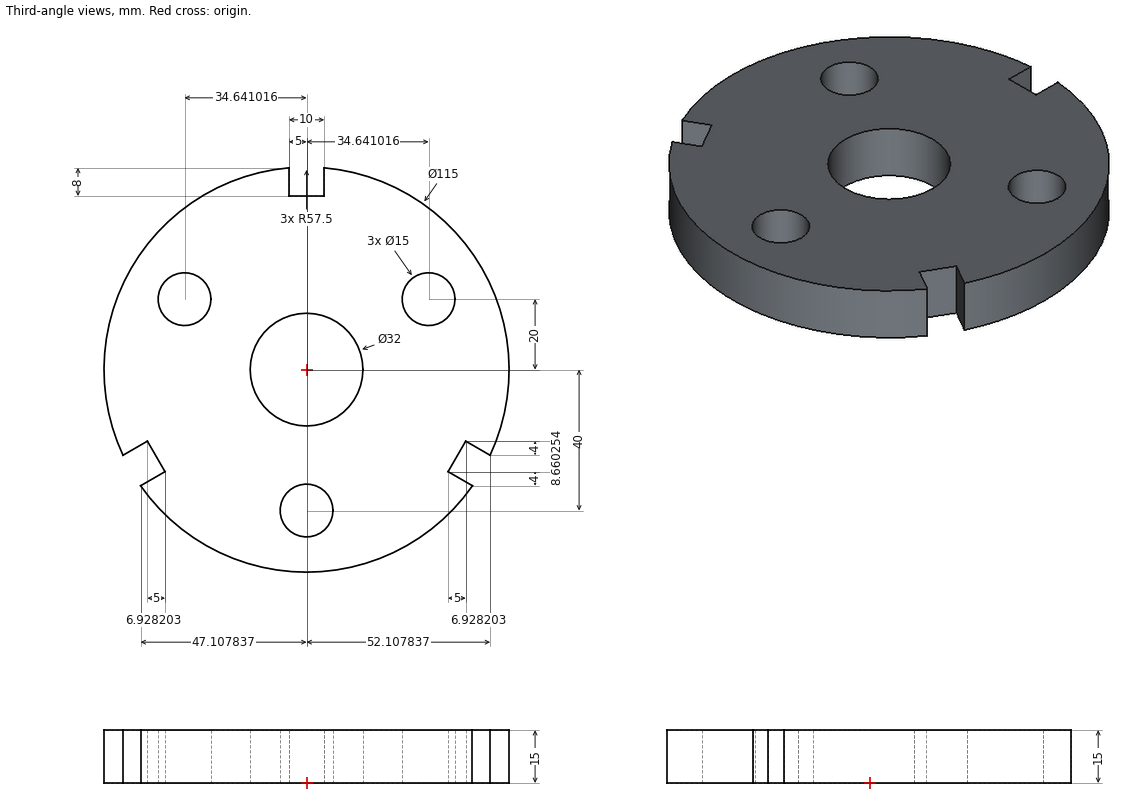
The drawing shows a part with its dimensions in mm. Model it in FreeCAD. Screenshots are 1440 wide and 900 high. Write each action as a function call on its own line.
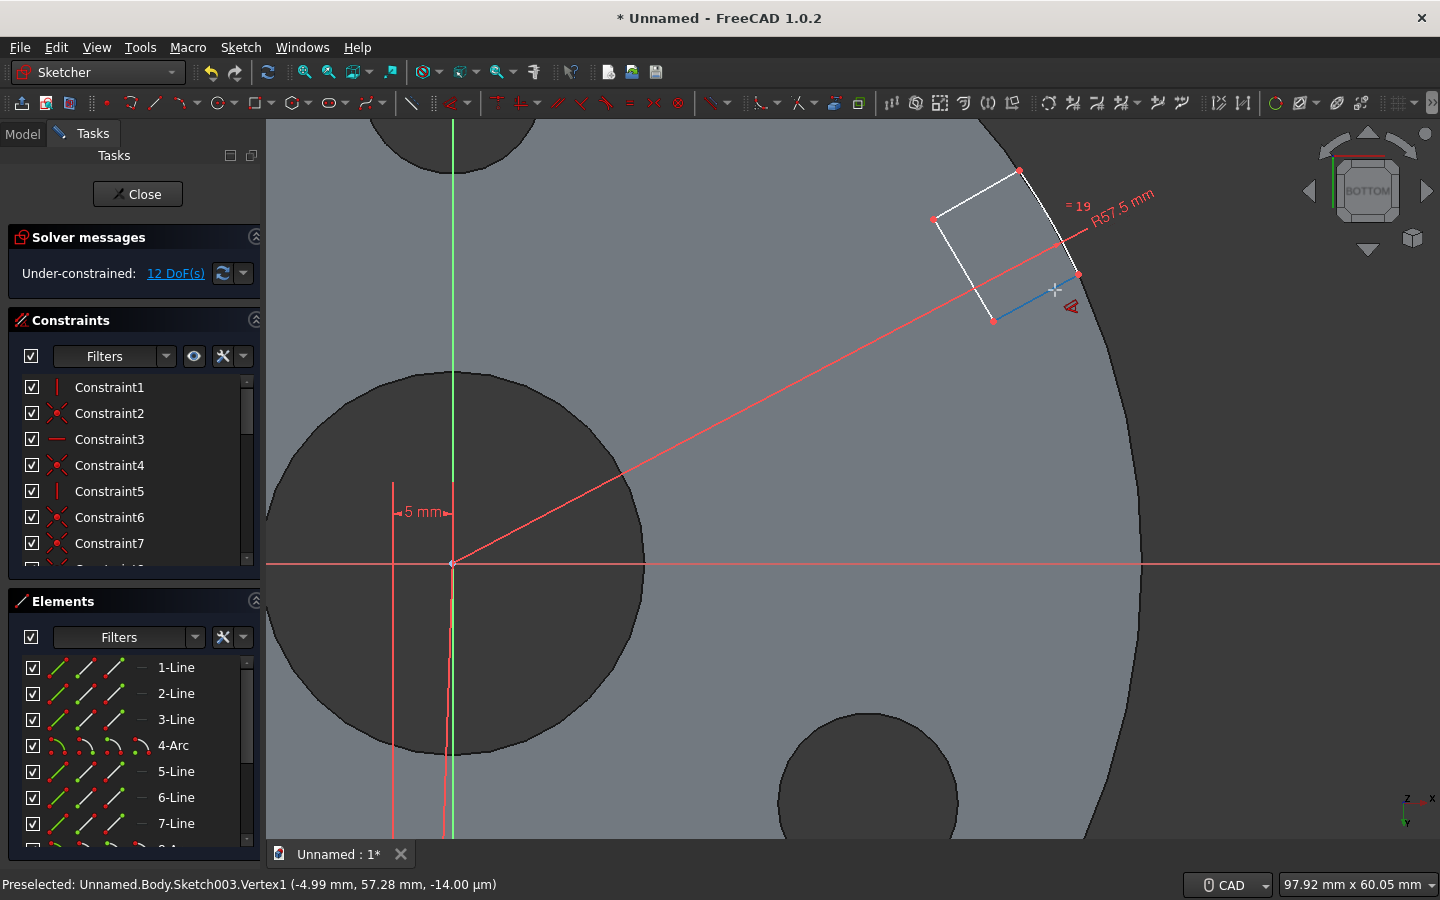
click(1053, 289)
click(1113, 298)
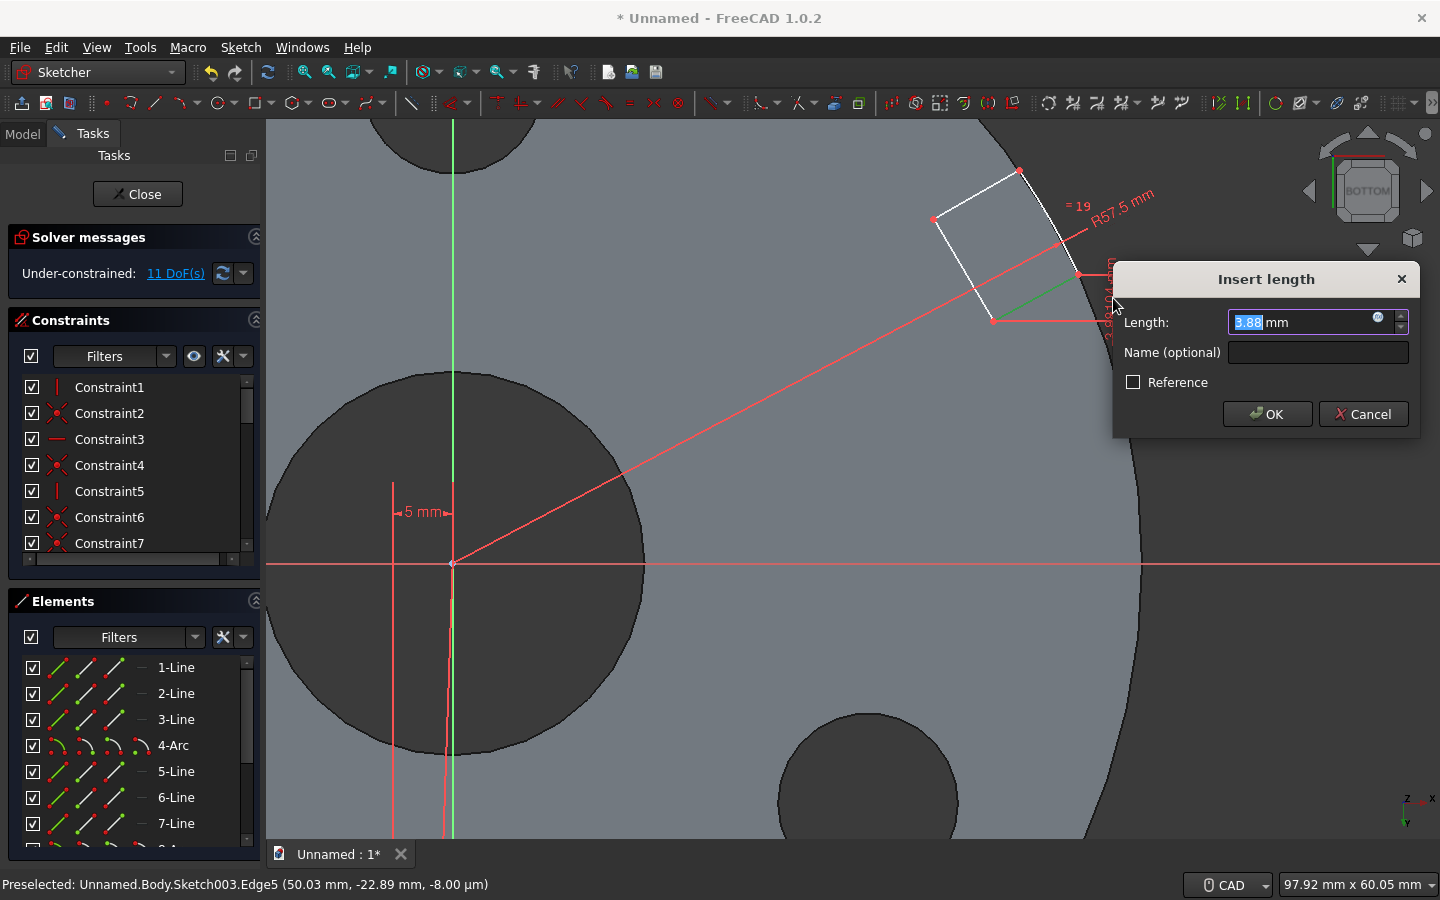
text(4)
key(Return)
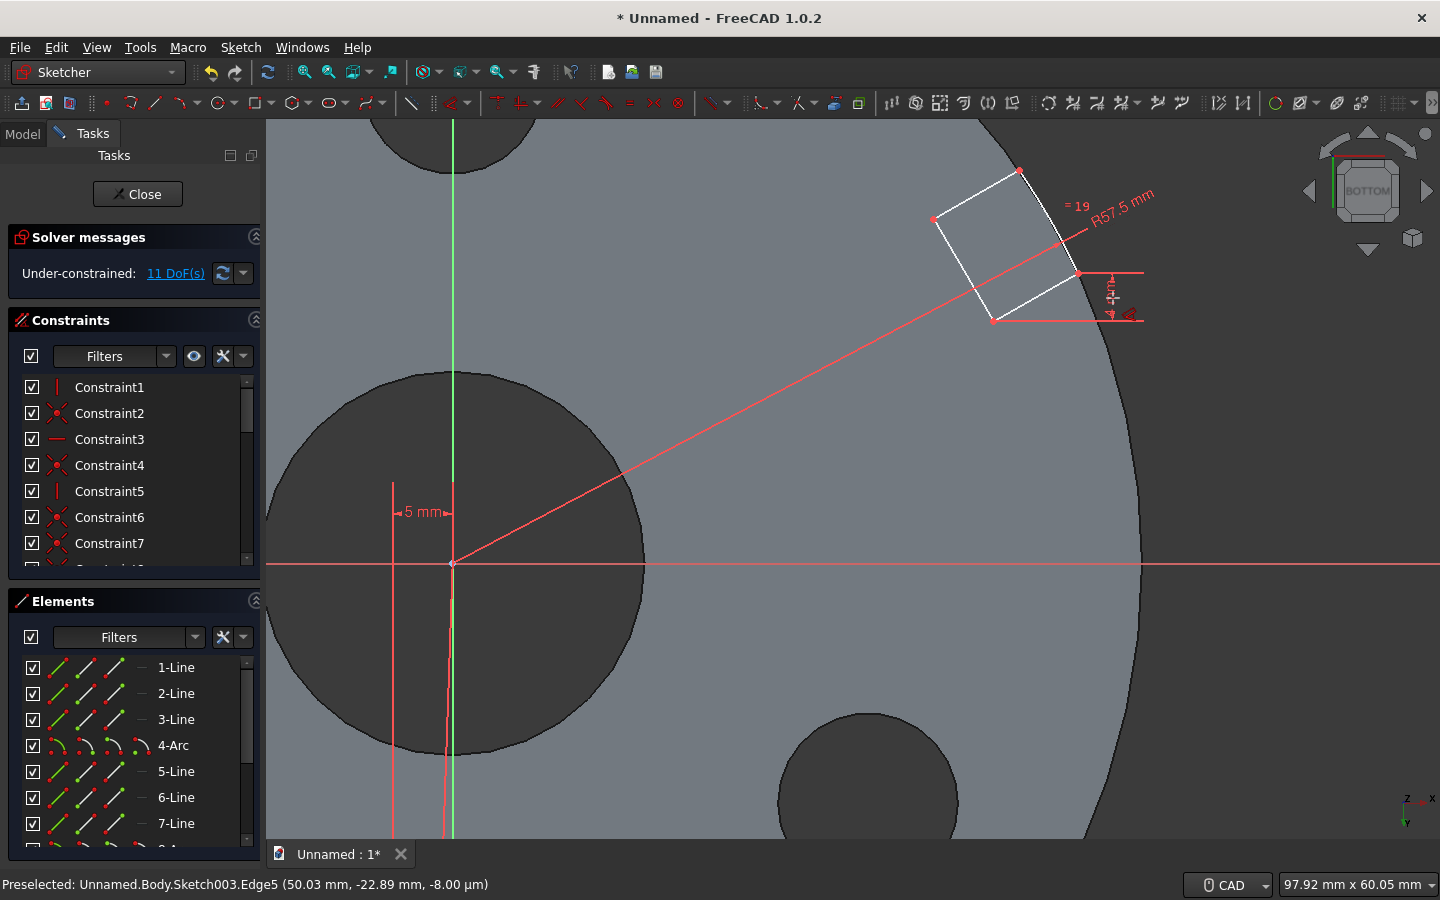
click(976, 291)
click(964, 185)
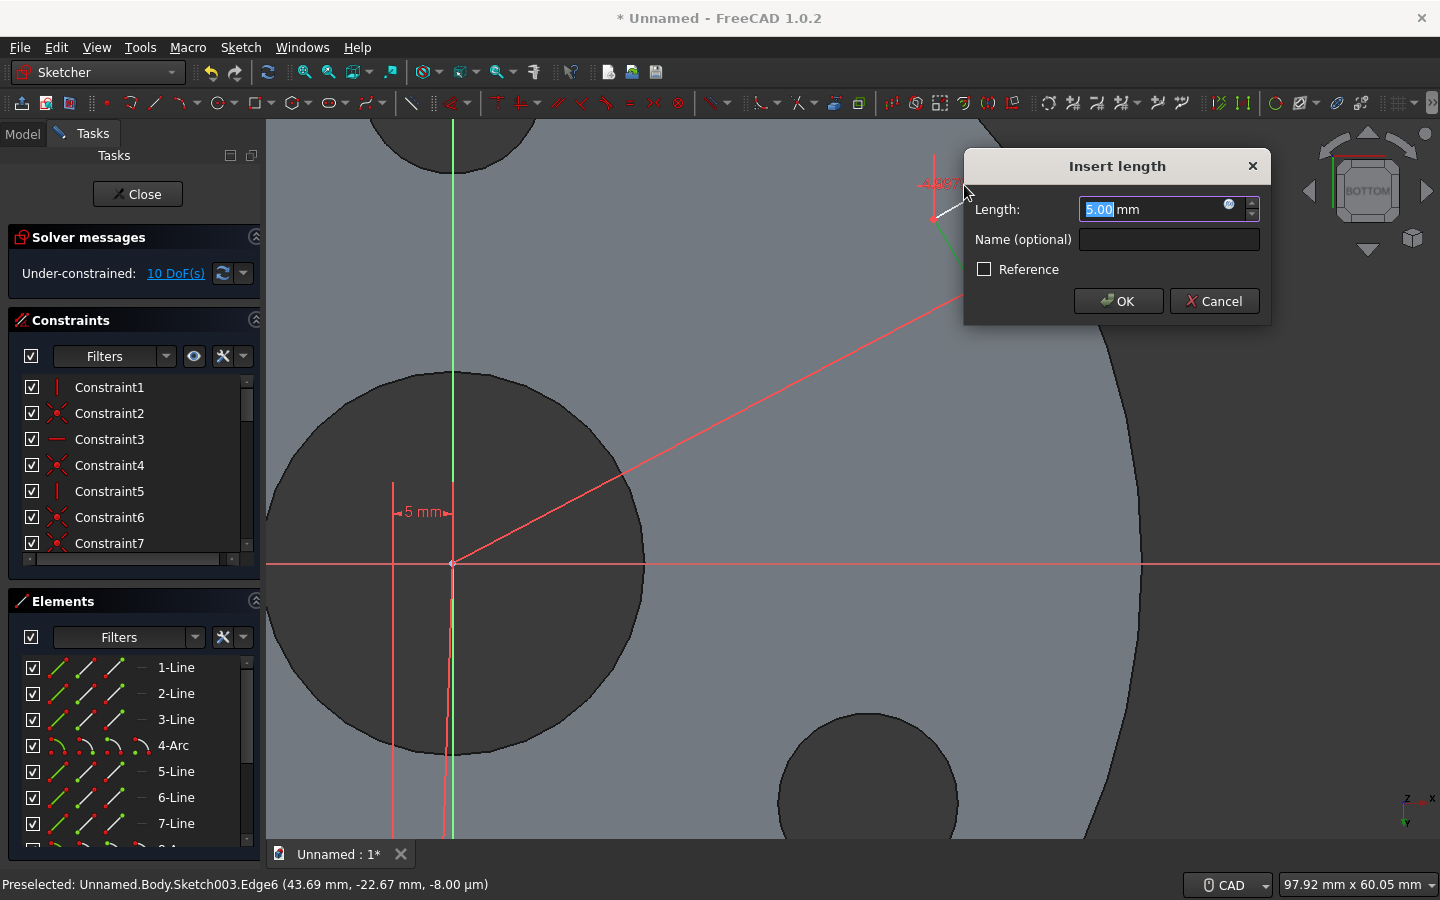
text(5)
key(Return)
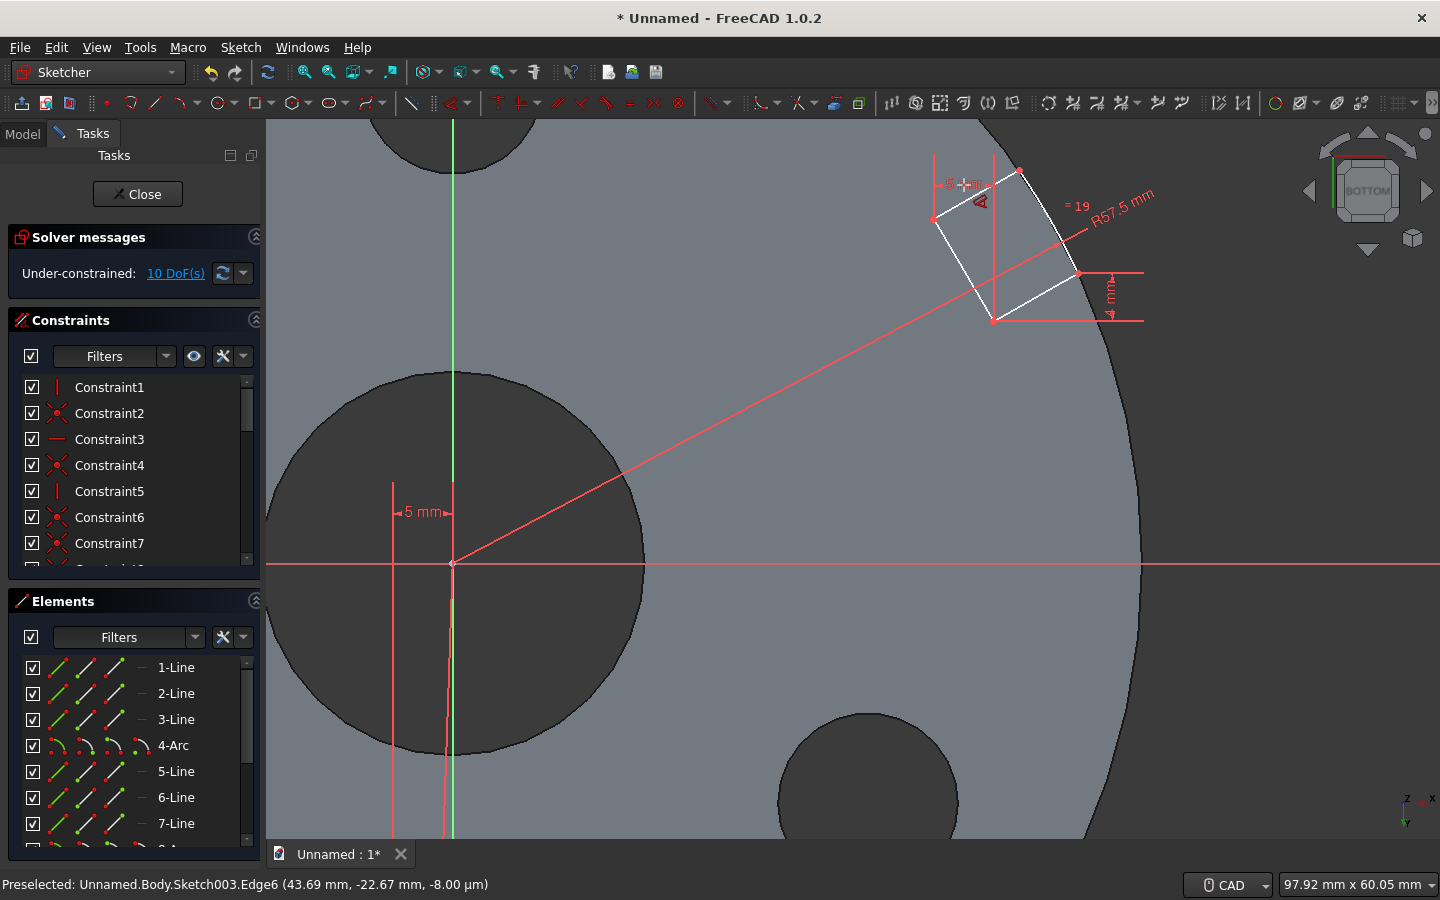
click(959, 204)
click(1053, 184)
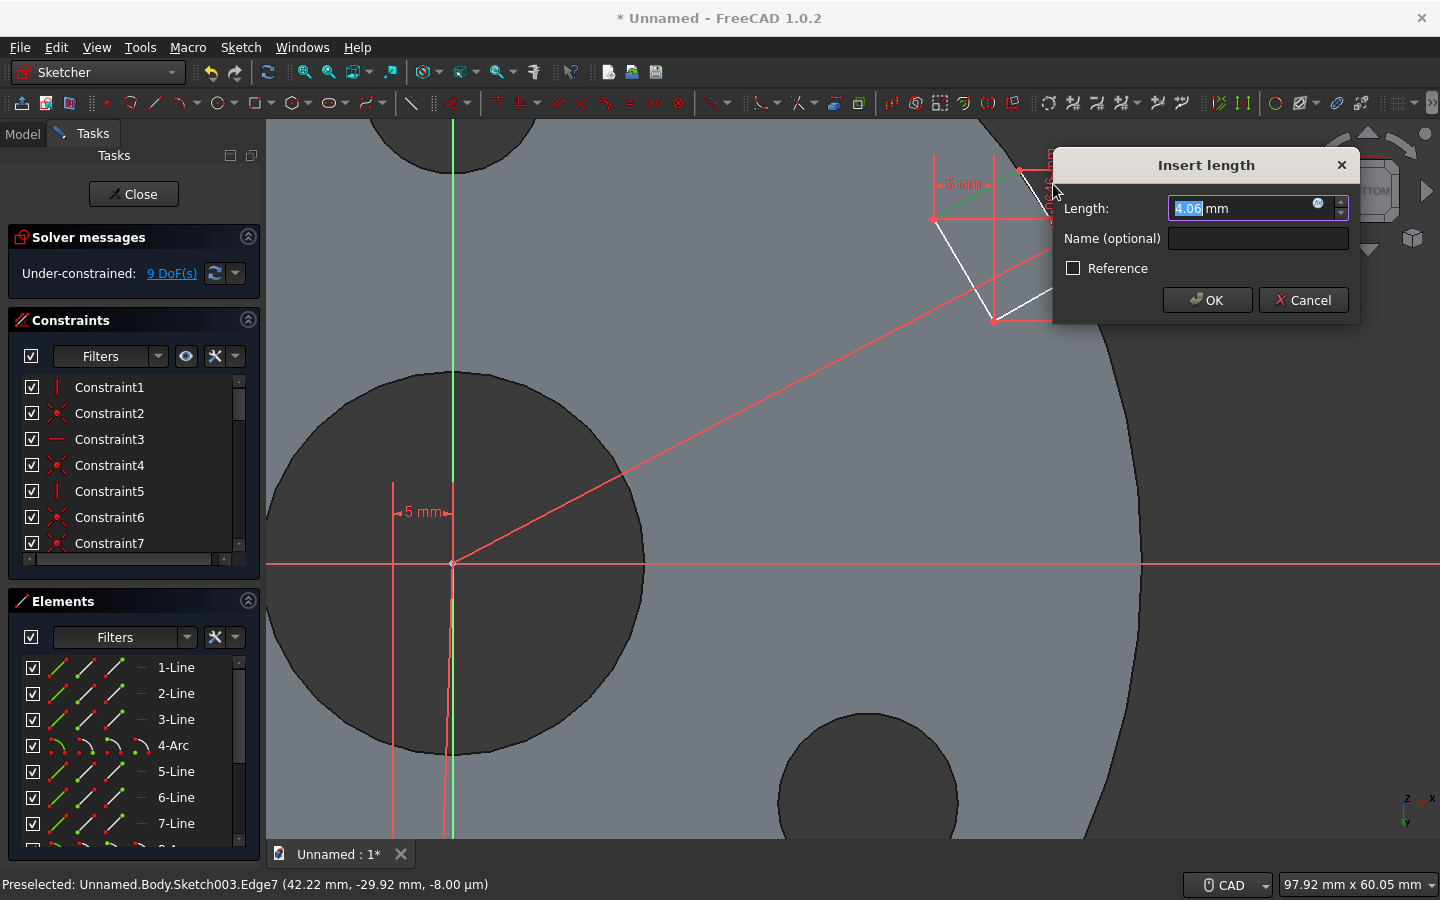
text(4)
key(Return)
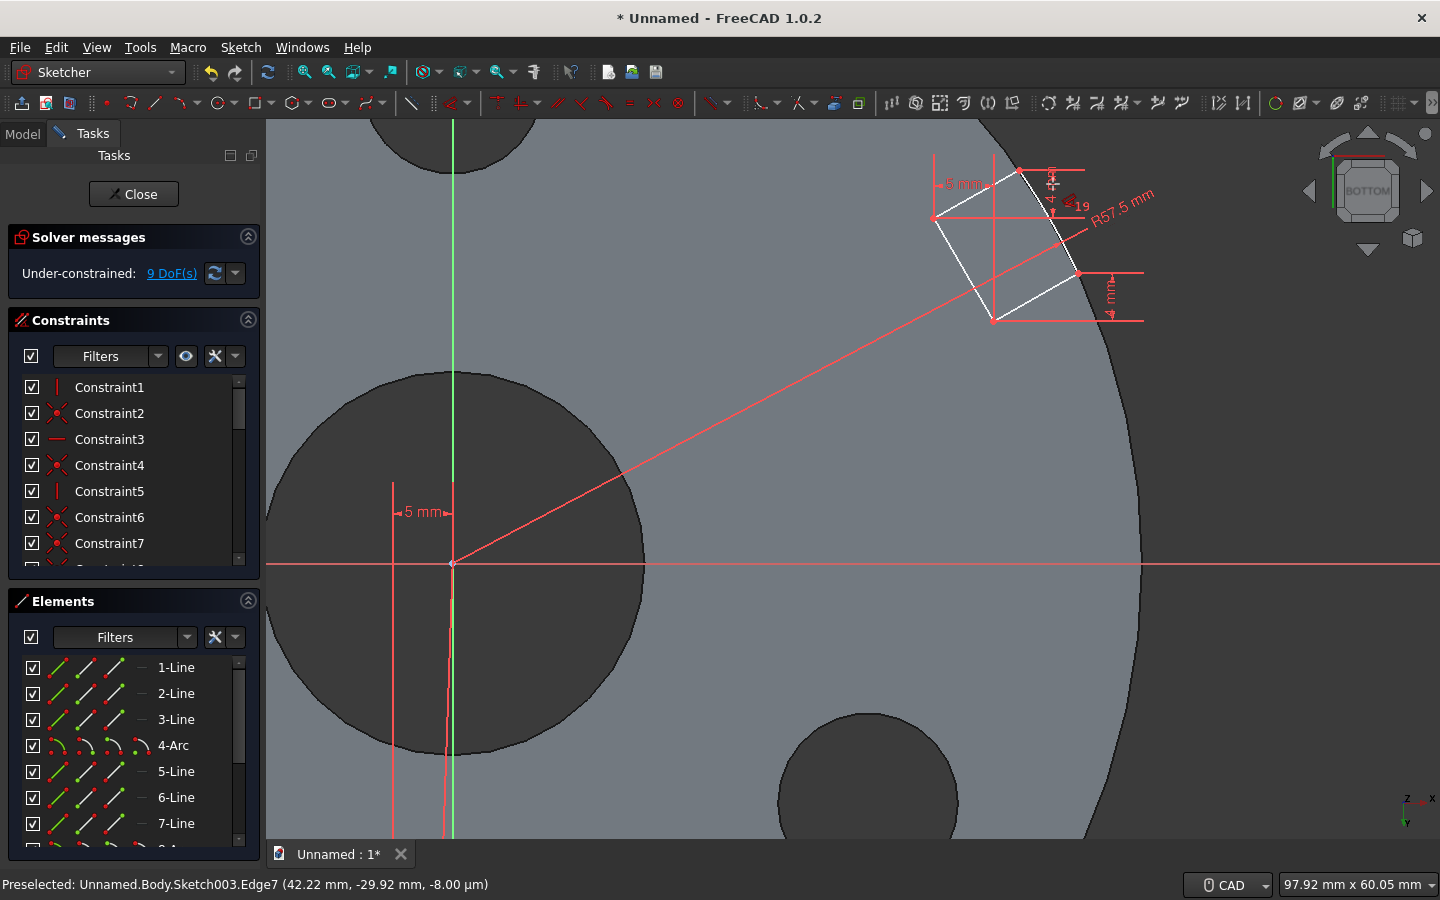
scroll(1055, 290, down, 4)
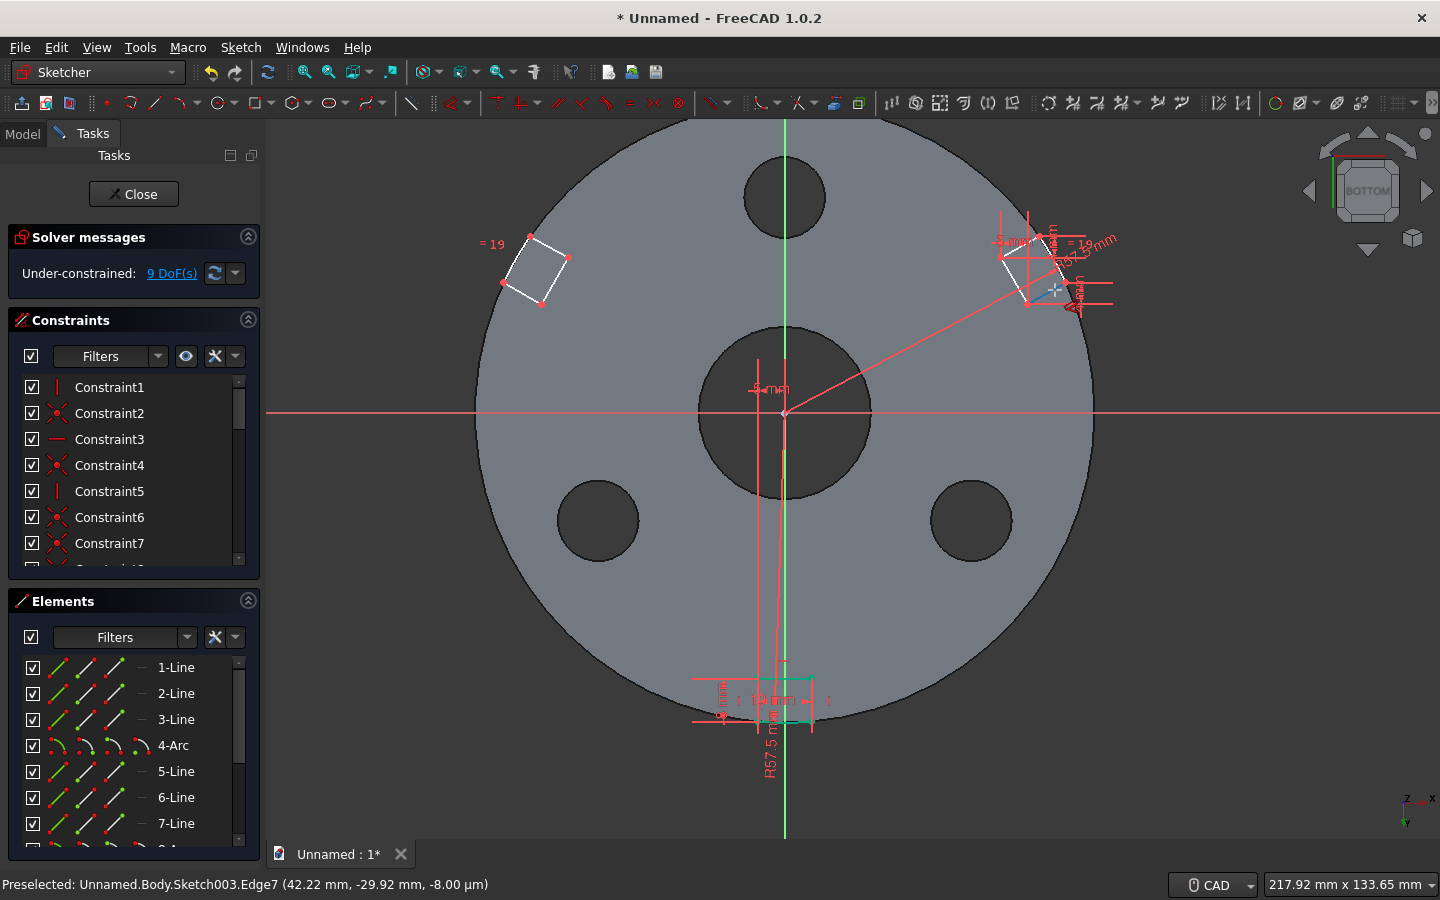
scroll(542, 243, up, 4)